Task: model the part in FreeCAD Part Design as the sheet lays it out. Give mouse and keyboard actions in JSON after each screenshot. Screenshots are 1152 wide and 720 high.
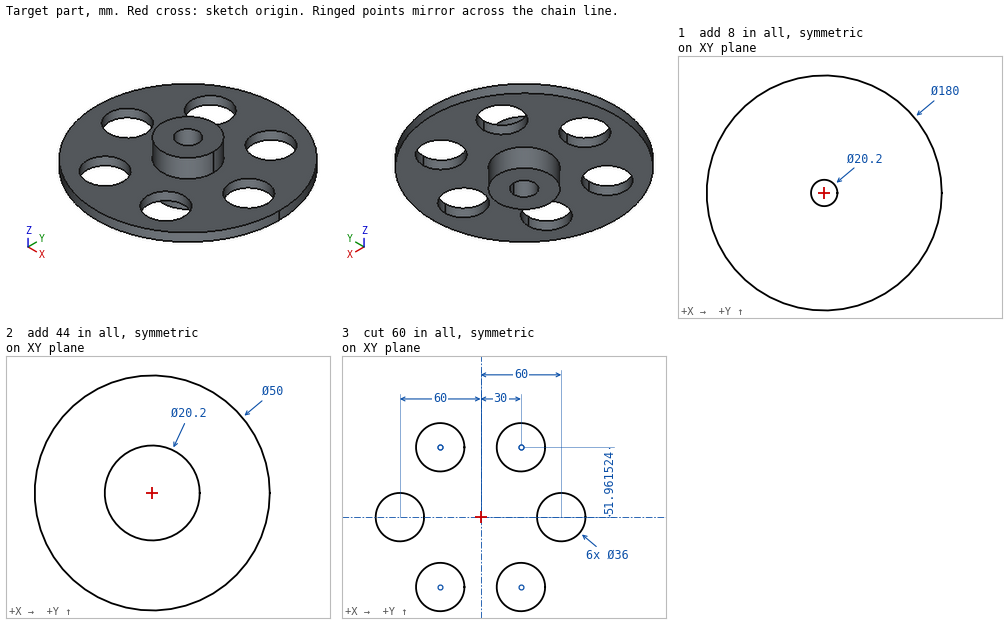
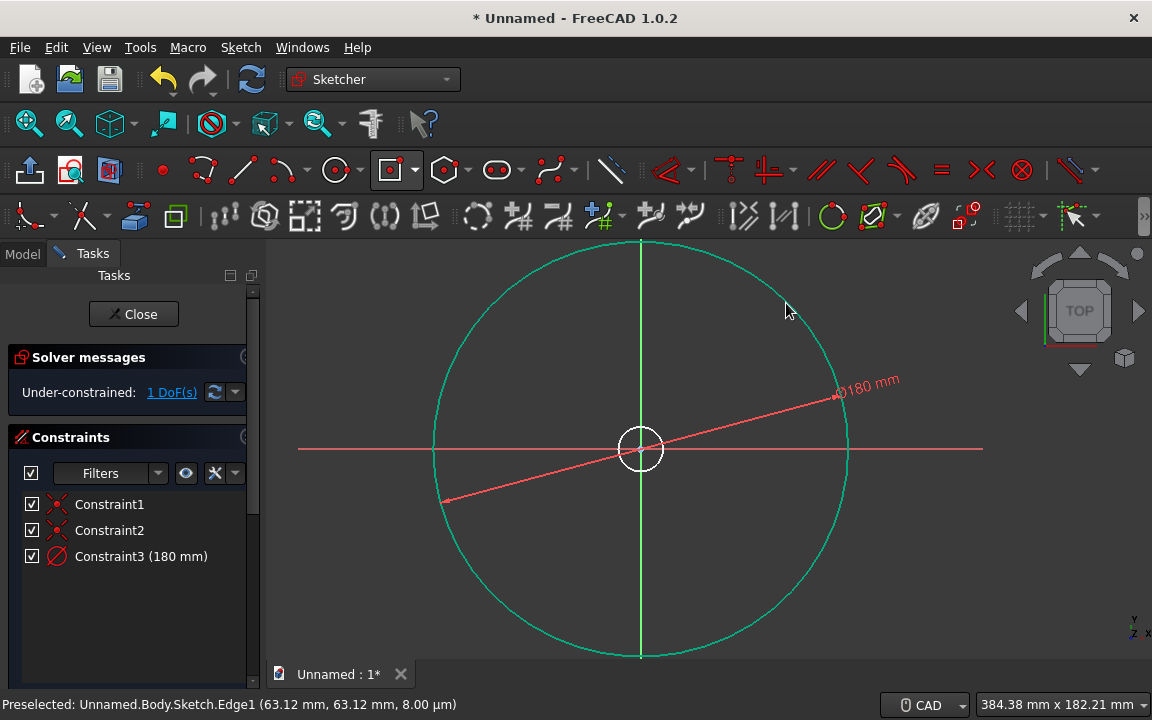
{"action": "left_click", "coordinate": [656, 433]}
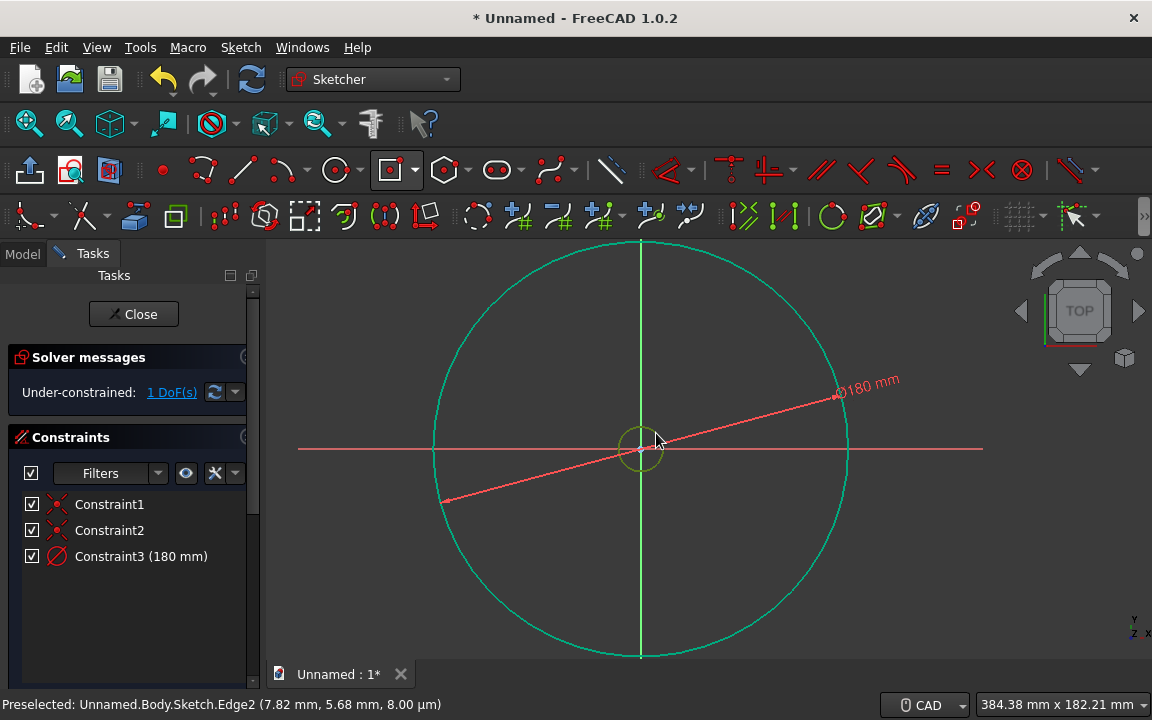
{"action": "key", "text": "k o"}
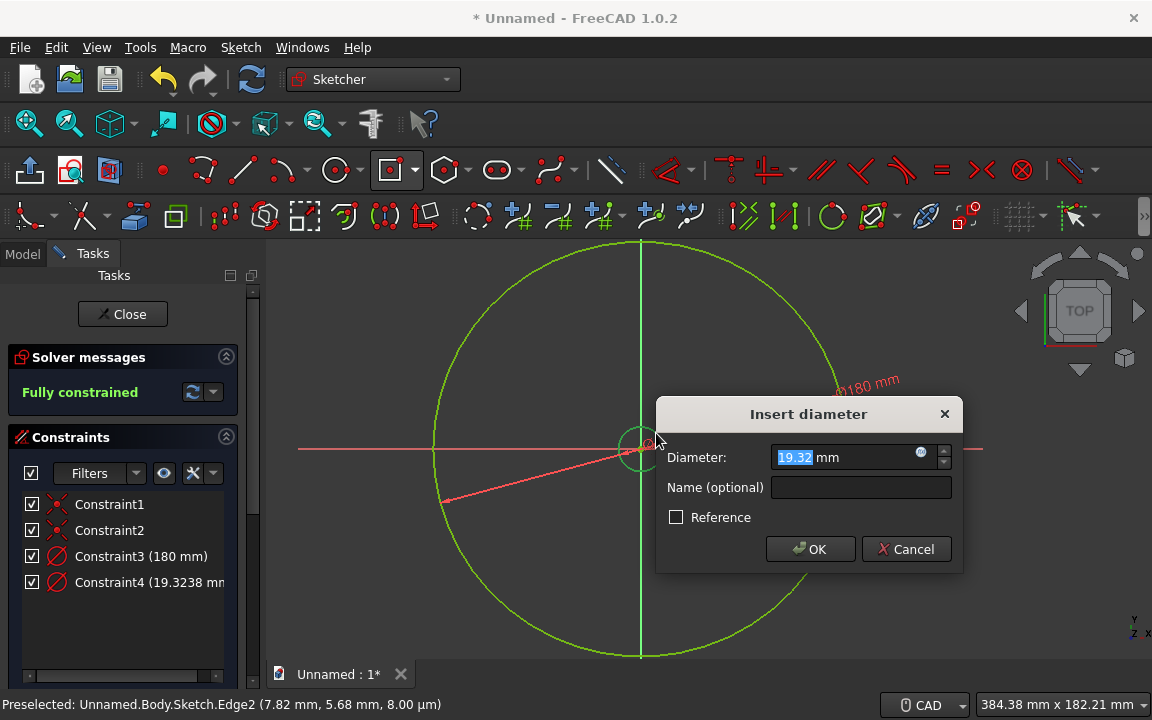
{"action": "type", "text": "20.2"}
{"action": "key", "text": "Return"}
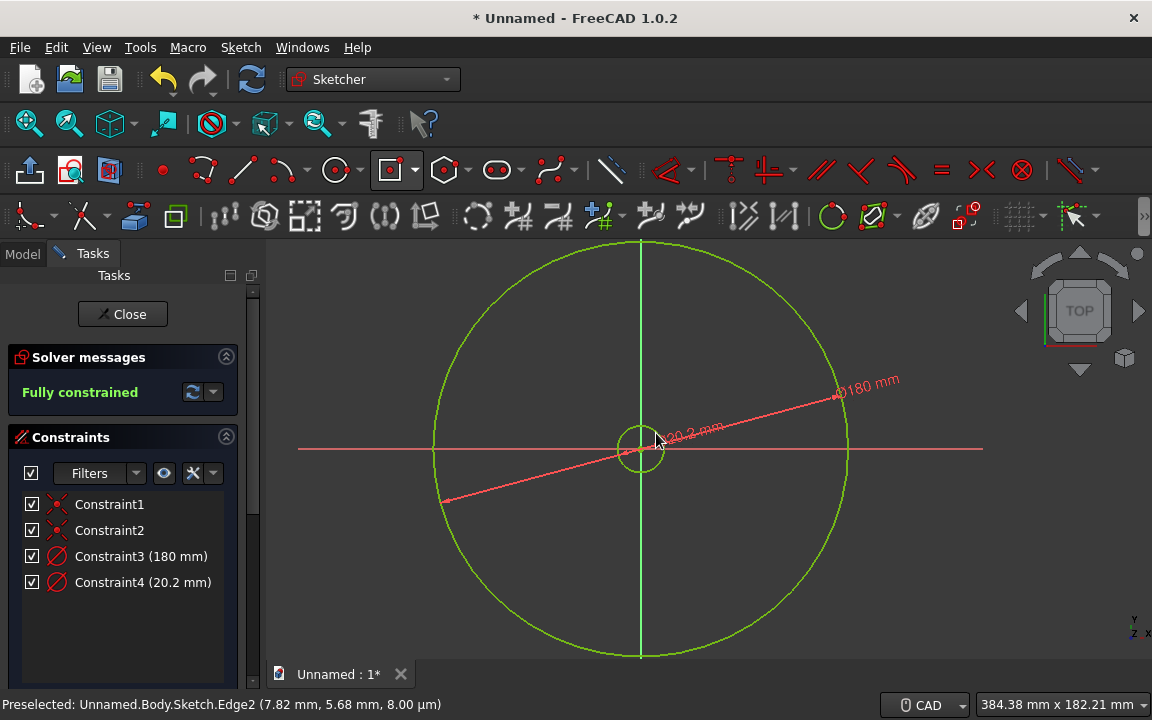
{"action": "left_click", "coordinate": [123, 314]}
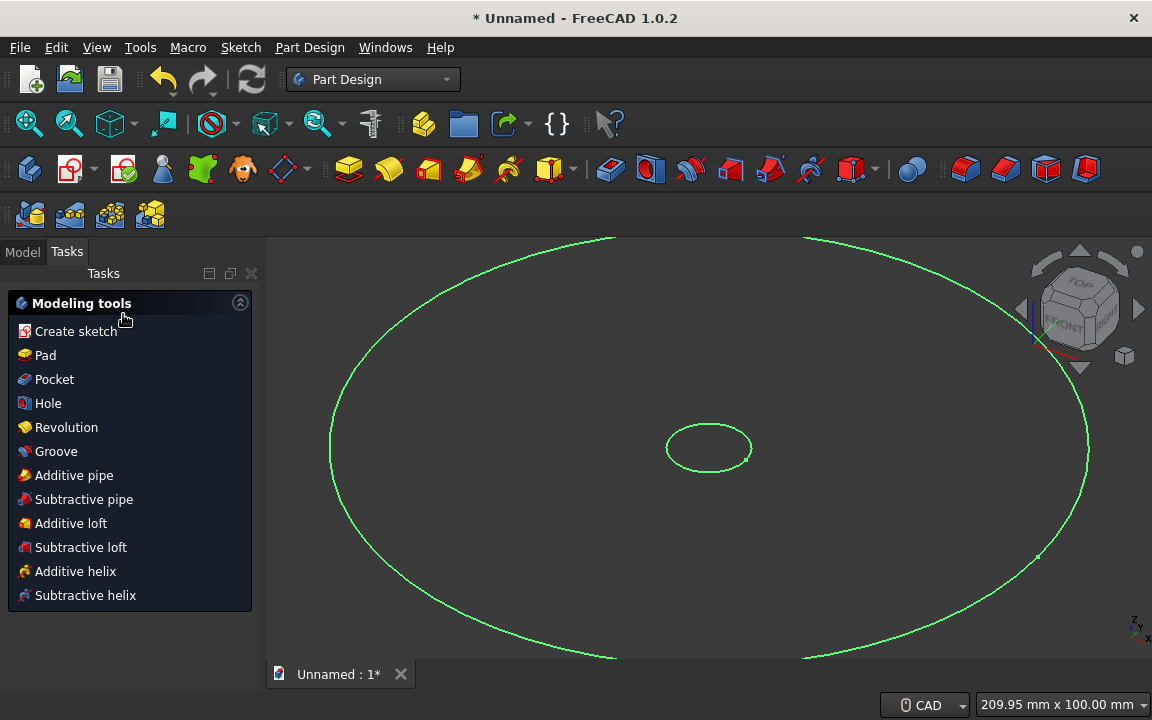
{"action": "left_click", "coordinate": [350, 170]}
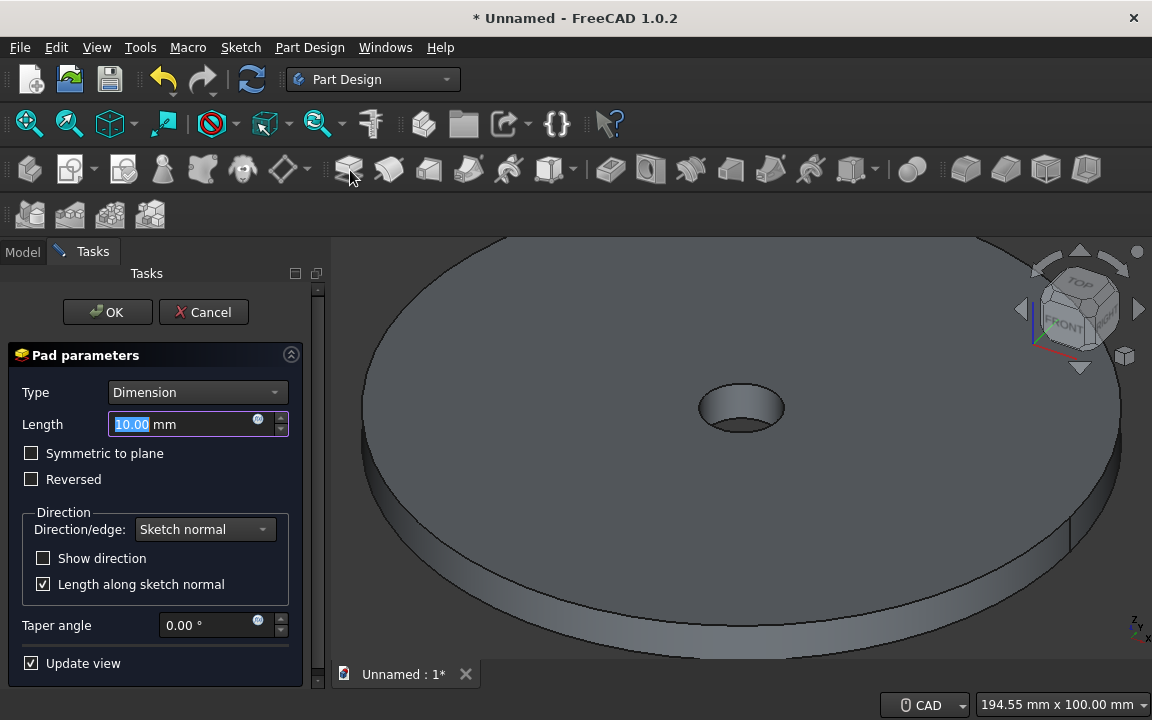
{"action": "type", "text": "8"}
{"action": "key", "text": "Tab"}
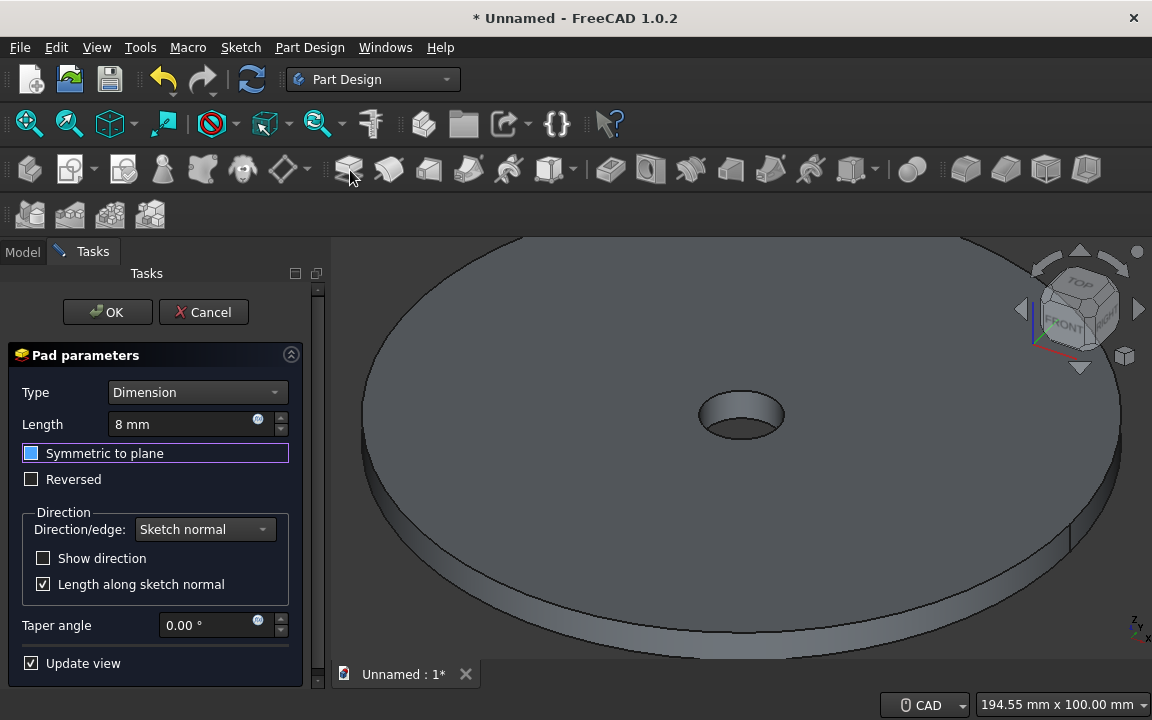
{"action": "left_click", "coordinate": [30, 453]}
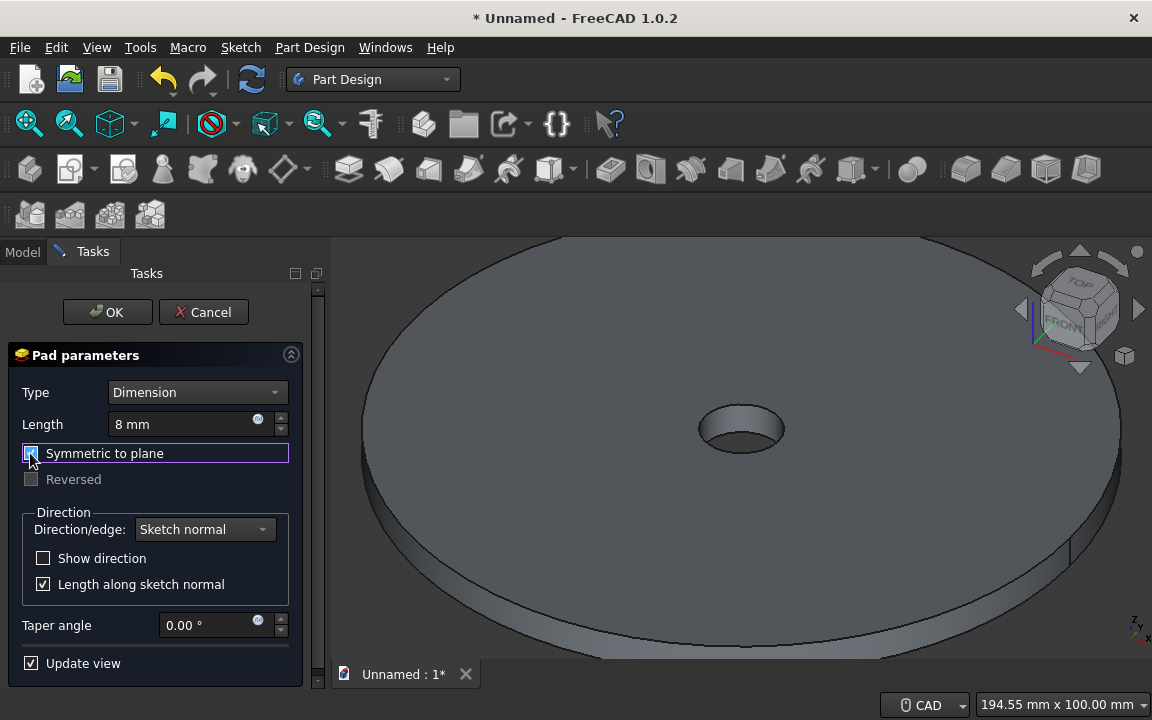
{"action": "left_click", "coordinate": [108, 312]}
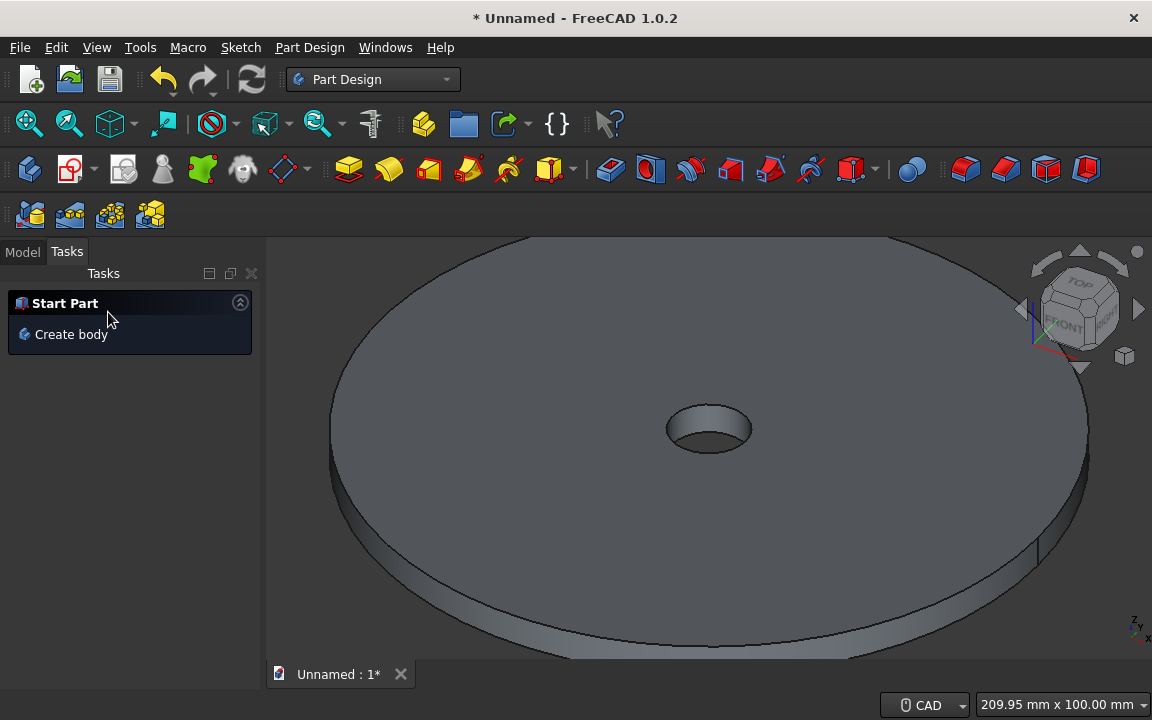
{"action": "left_click", "coordinate": [30, 124]}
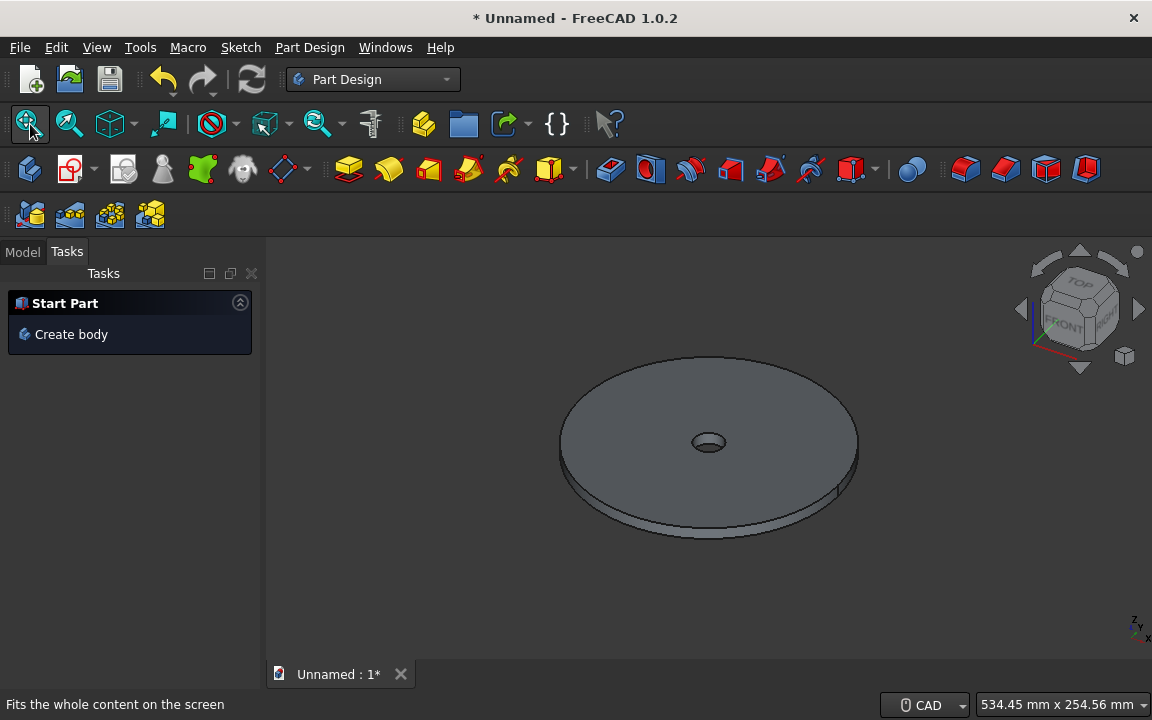
{"action": "left_click", "coordinate": [70, 170]}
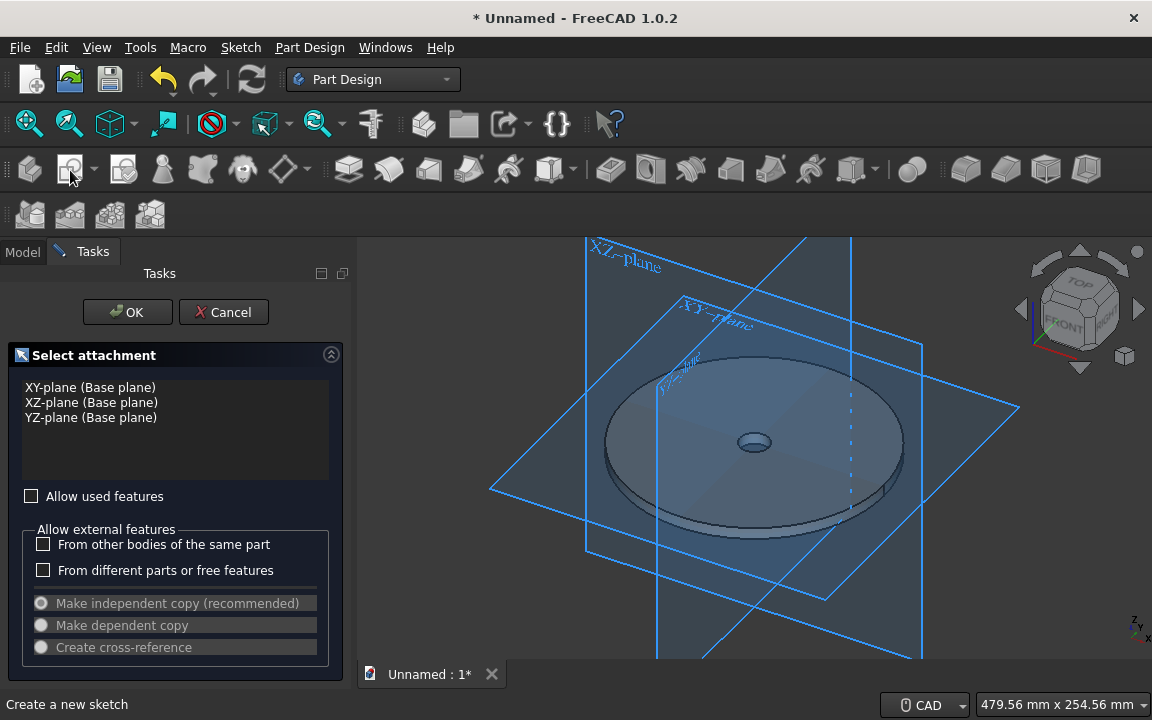
{"action": "left_click", "coordinate": [82, 388]}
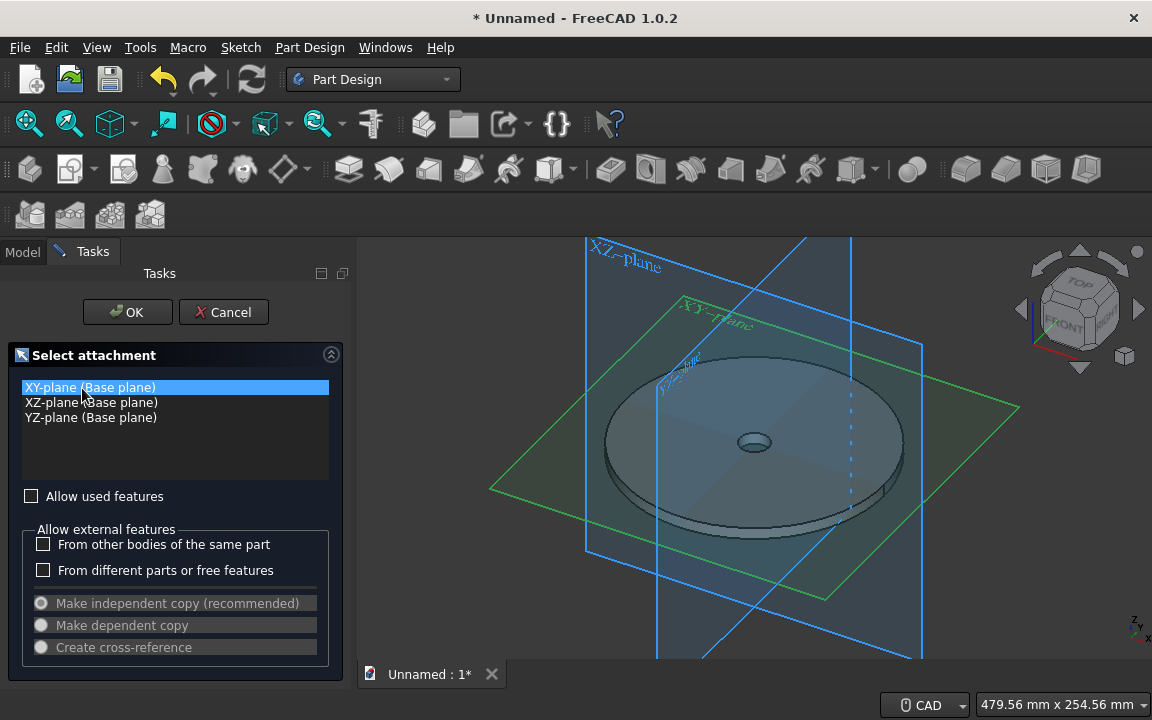
{"action": "left_click", "coordinate": [128, 312]}